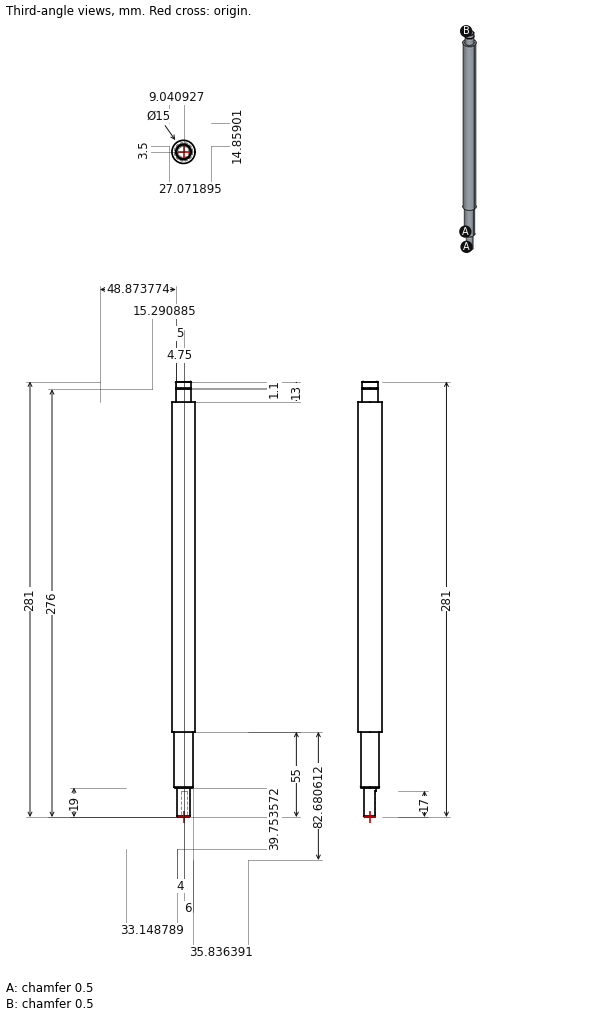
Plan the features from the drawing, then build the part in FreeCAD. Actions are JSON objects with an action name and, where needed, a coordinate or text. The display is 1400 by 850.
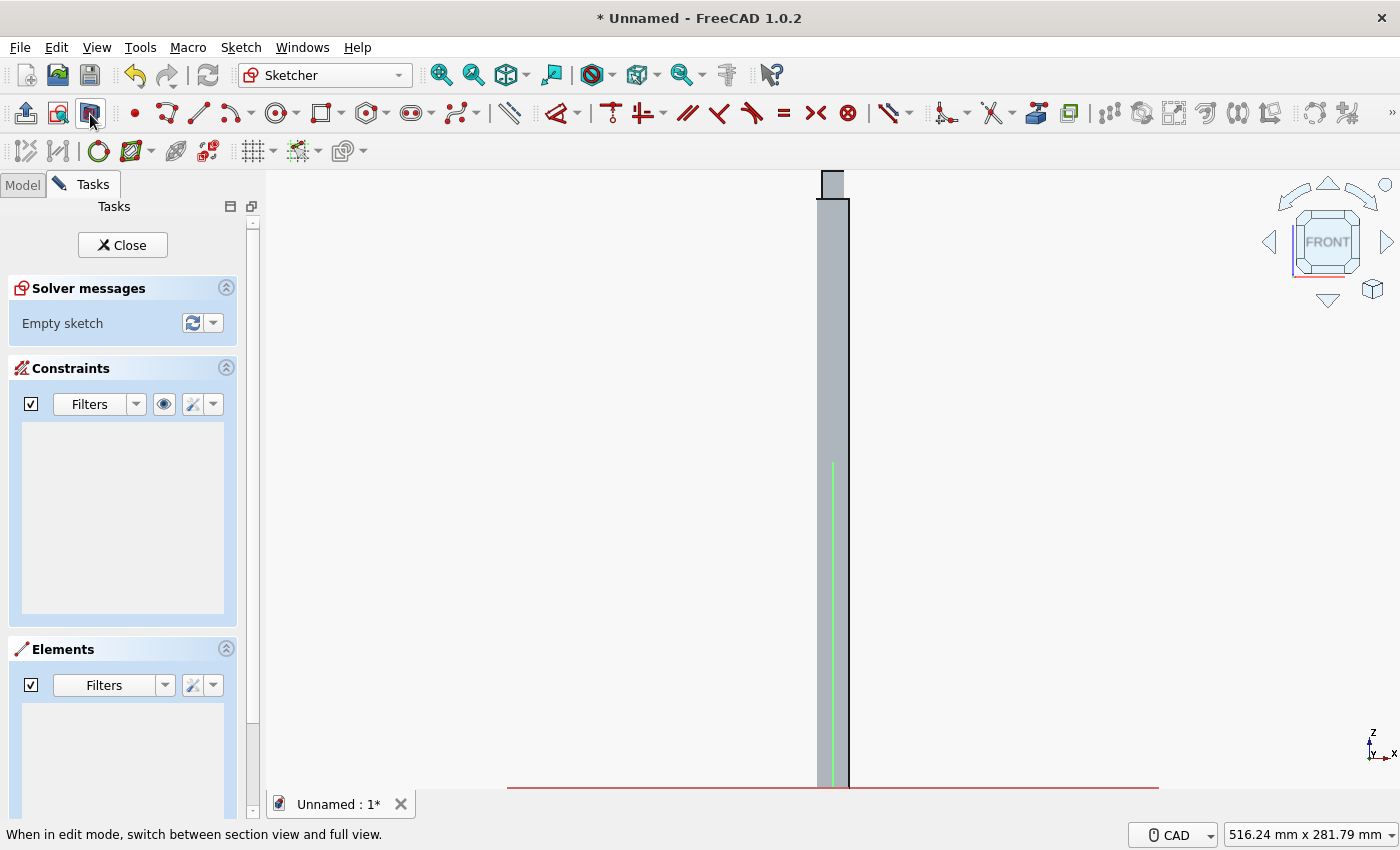
{"action": "scroll", "coordinate": [764, 480], "scroll_direction": "down", "scroll_amount": 5}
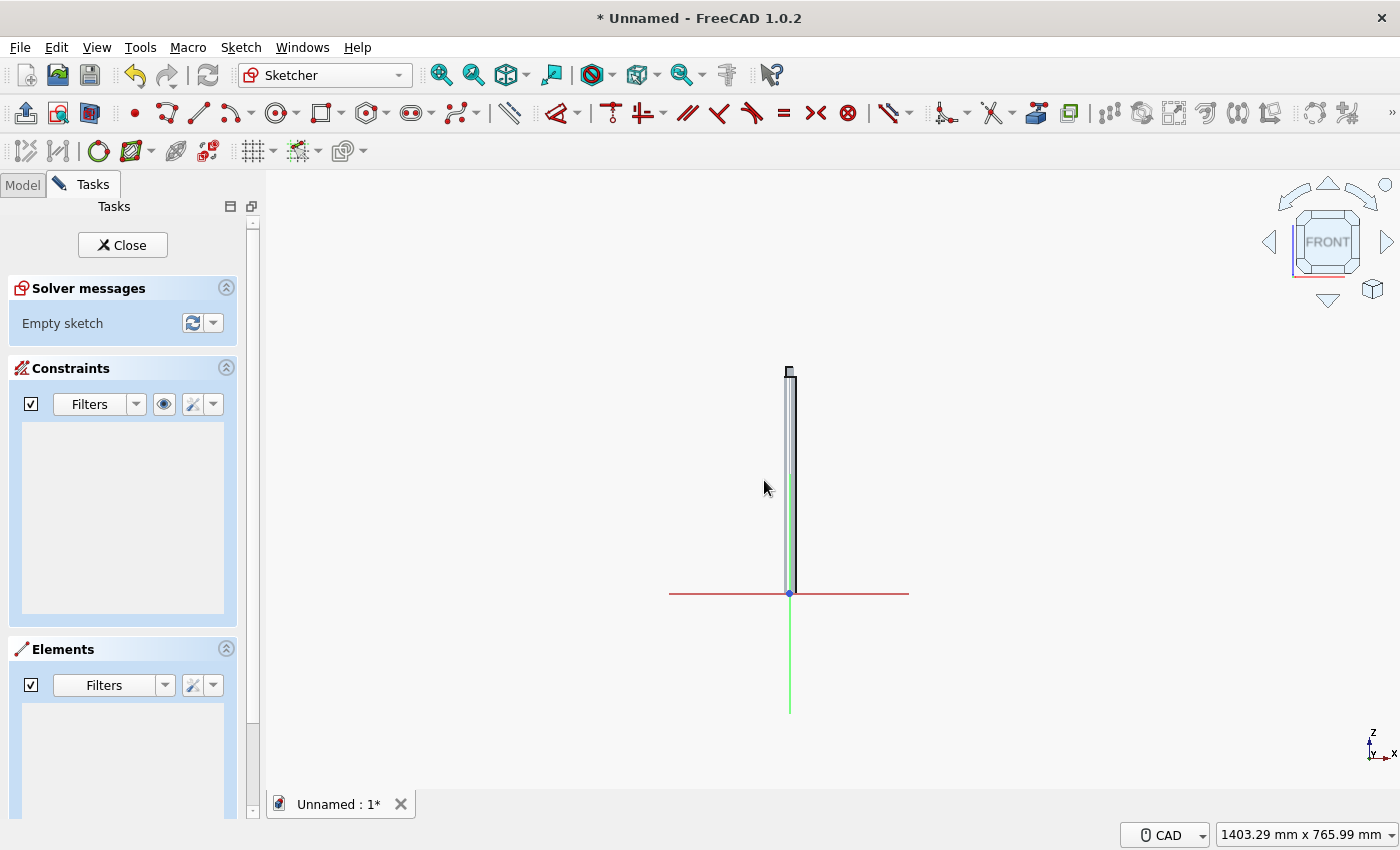
{"action": "scroll", "coordinate": [815, 603], "scroll_direction": "up", "scroll_amount": 9}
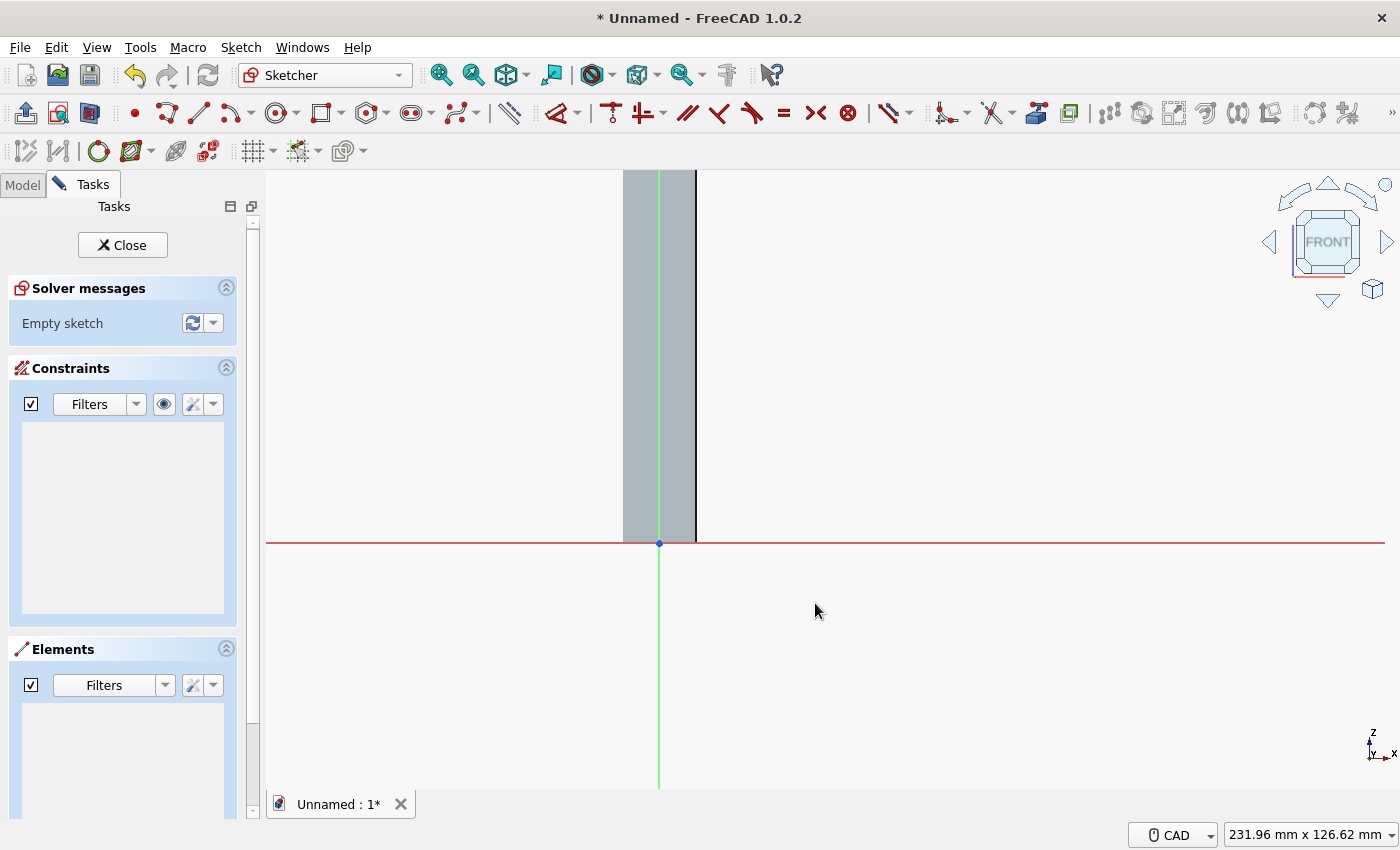
{"action": "left_click", "coordinate": [322, 114]}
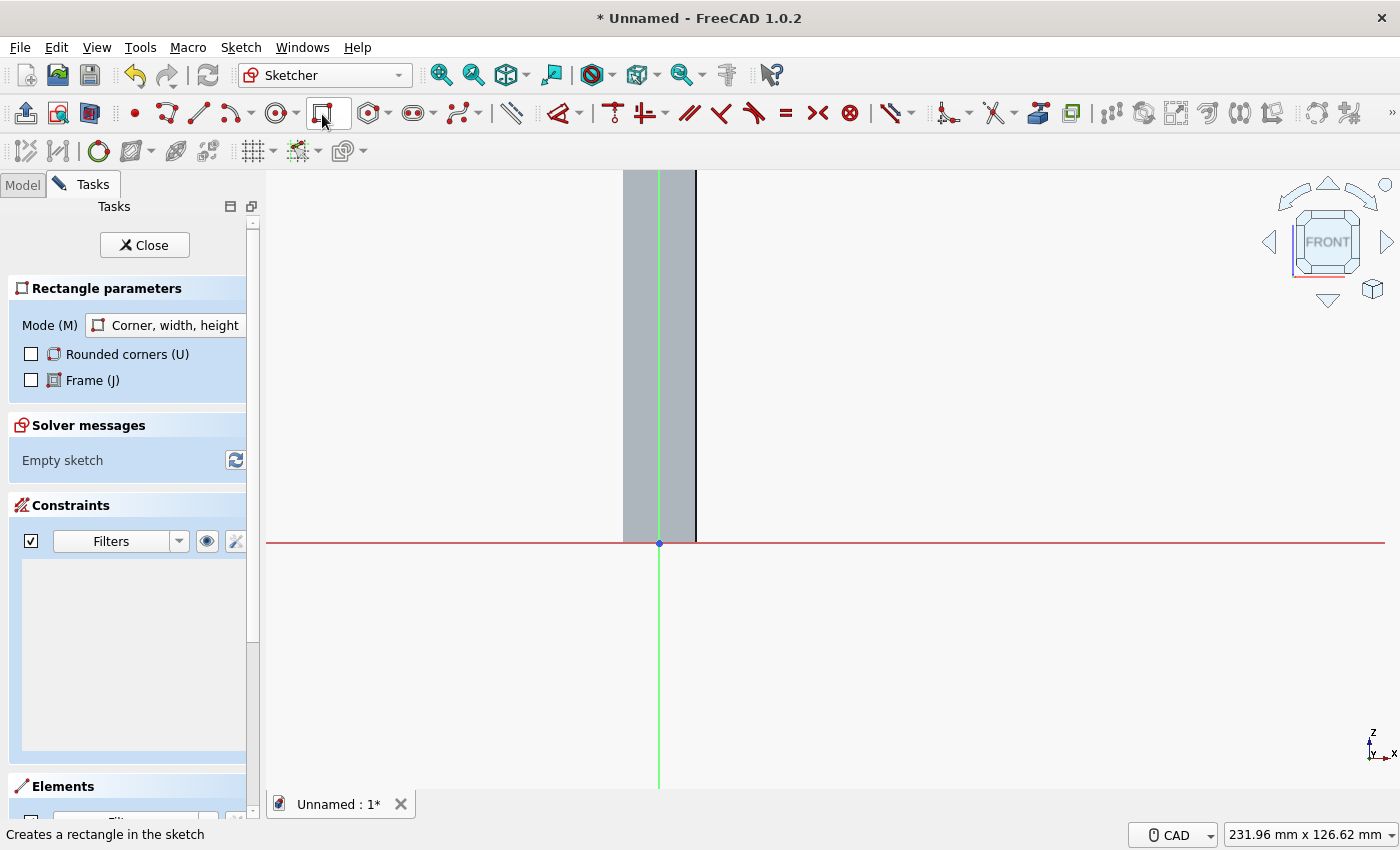
{"action": "left_click", "coordinate": [689, 274]}
{"action": "mouse_move", "coordinate": [864, 678]}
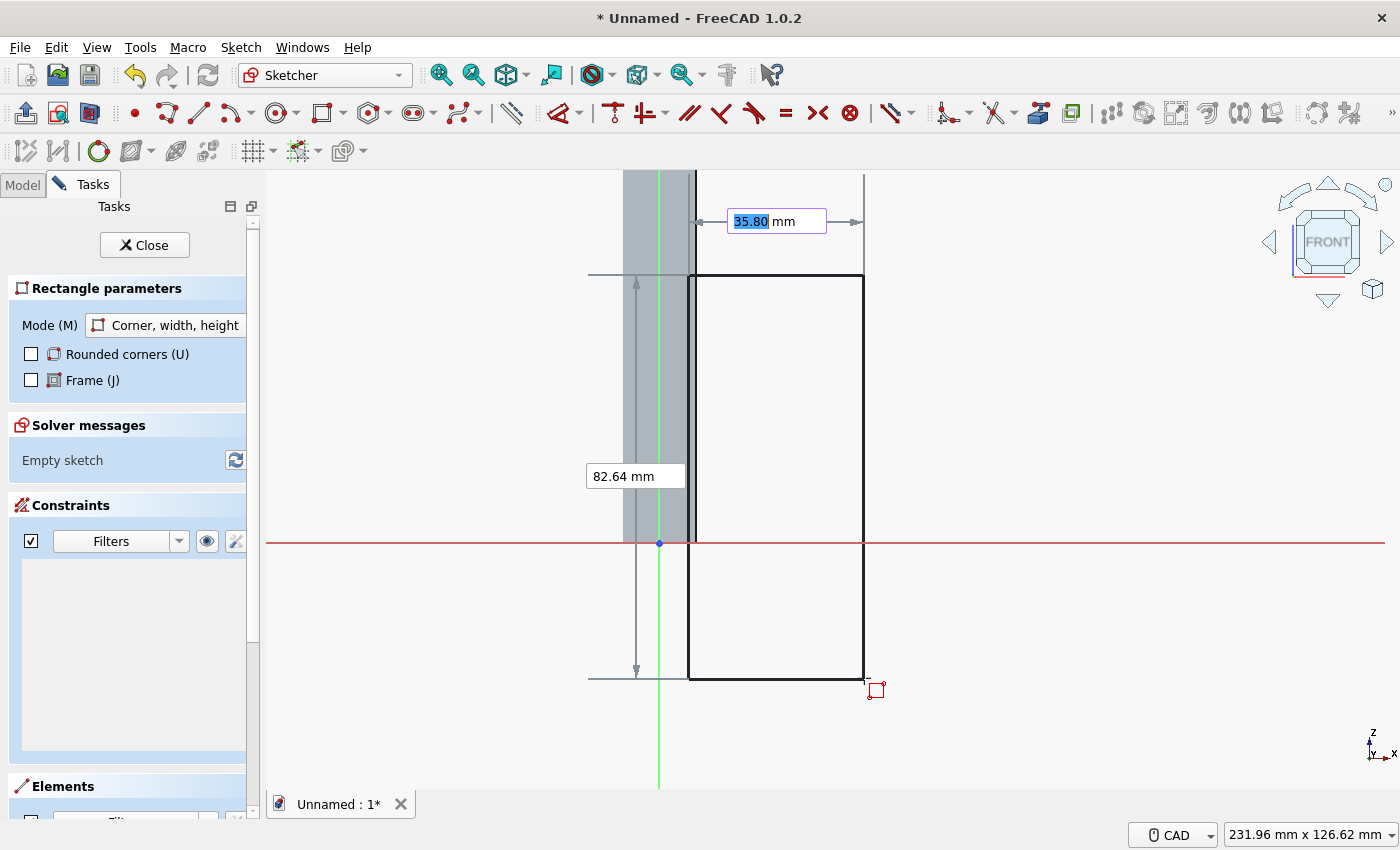
{"action": "type", "text": "35.836391"}
{"action": "key", "text": "Tab"}
{"action": "type", "text": "82.680612"}
{"action": "key", "text": "Return"}
{"action": "key", "text": "Escape"}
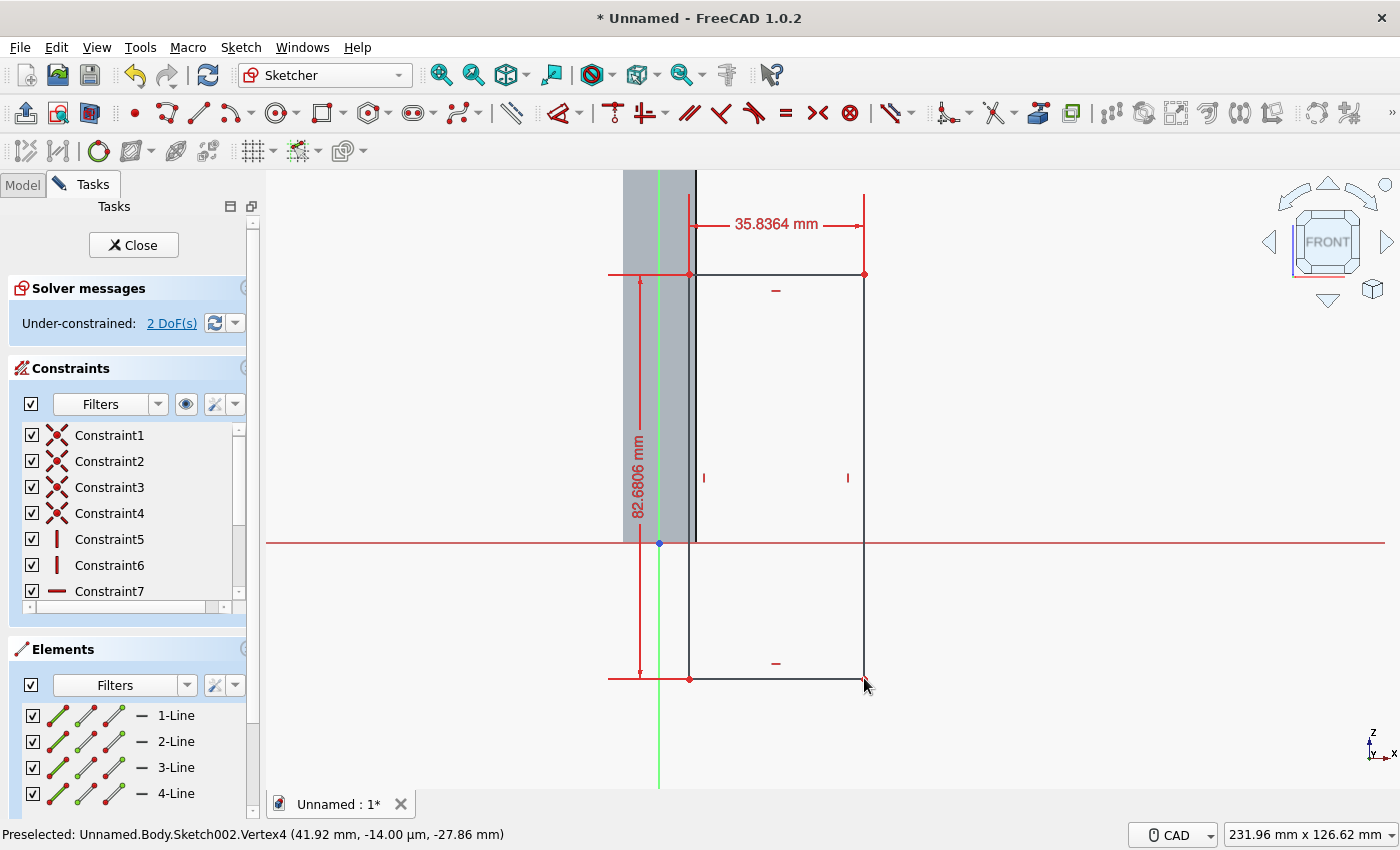
{"action": "left_click", "coordinate": [558, 114]}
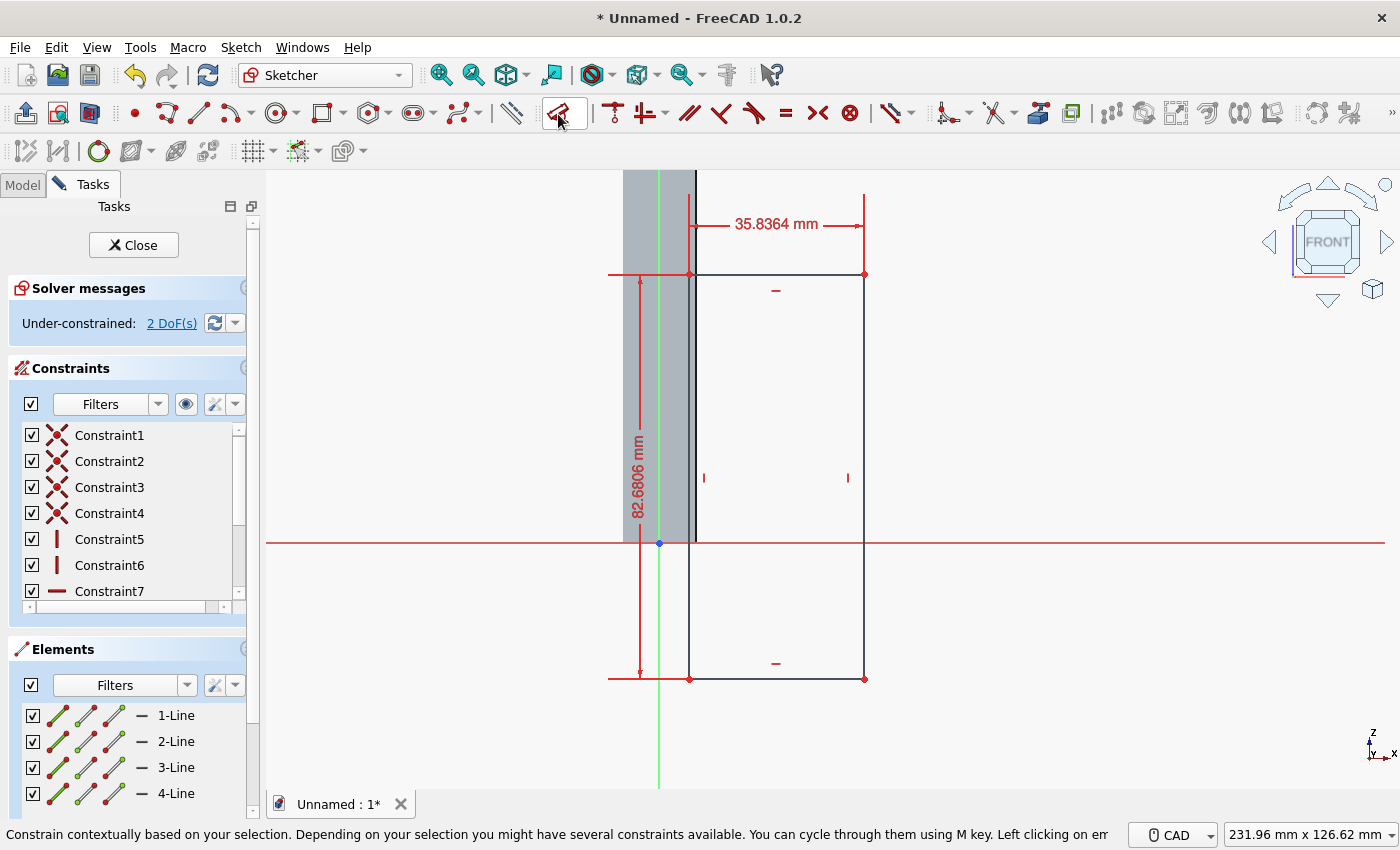
{"action": "scroll", "coordinate": [689, 275], "scroll_direction": "up", "scroll_amount": 2}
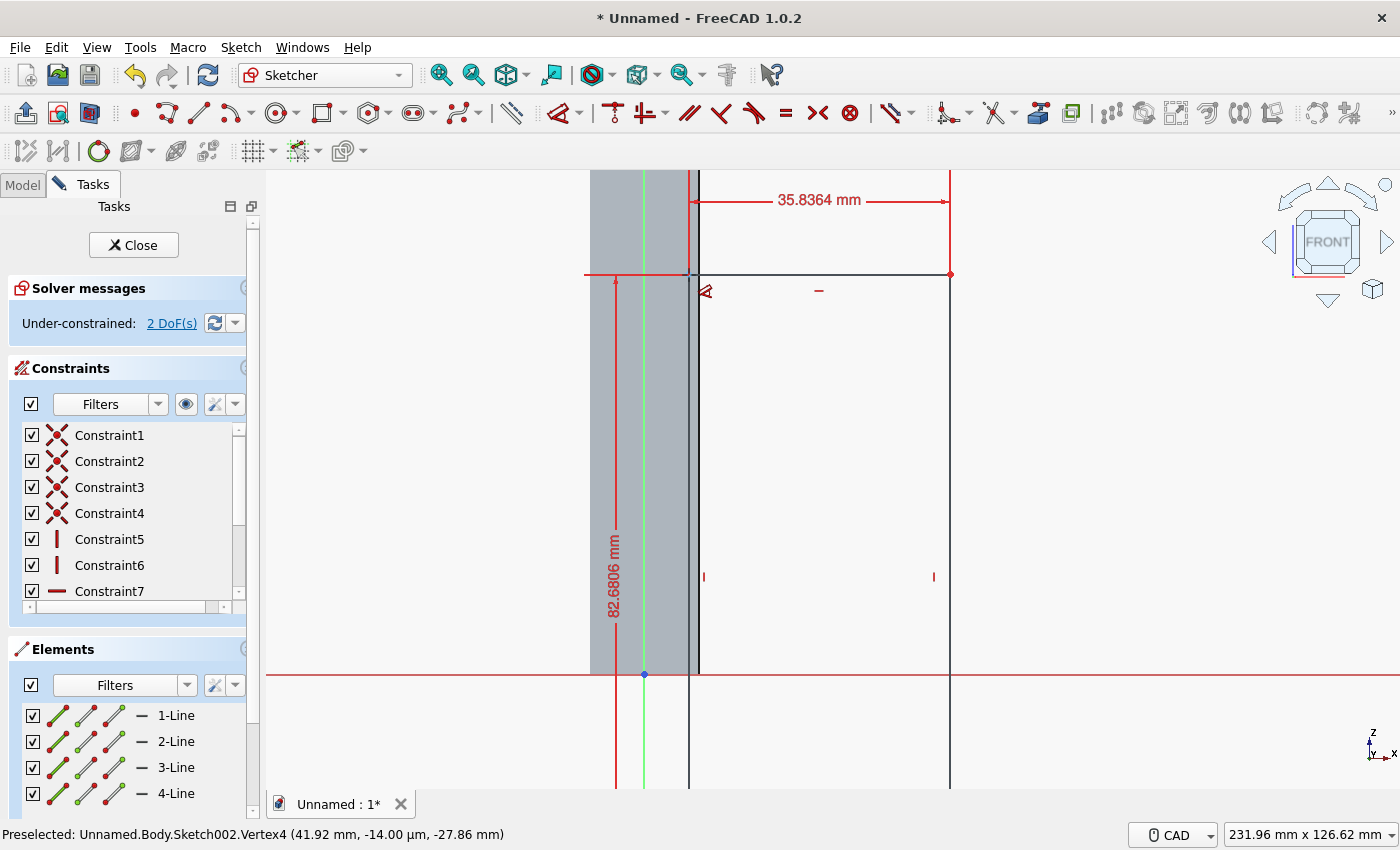
{"action": "left_click", "coordinate": [689, 275]}
{"action": "left_click", "coordinate": [667, 241]}